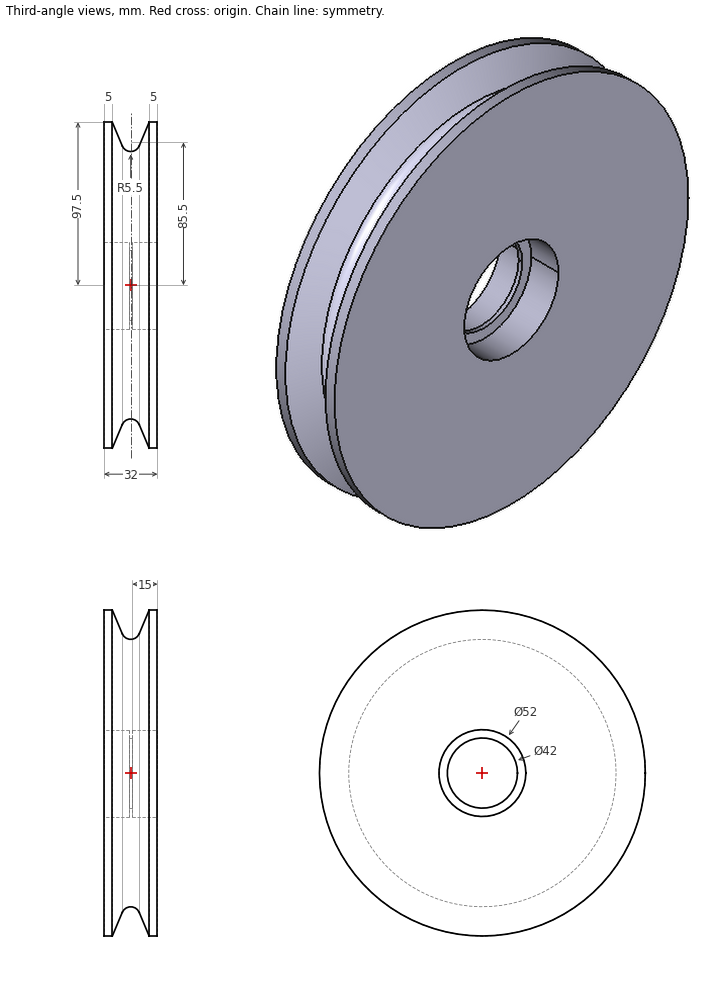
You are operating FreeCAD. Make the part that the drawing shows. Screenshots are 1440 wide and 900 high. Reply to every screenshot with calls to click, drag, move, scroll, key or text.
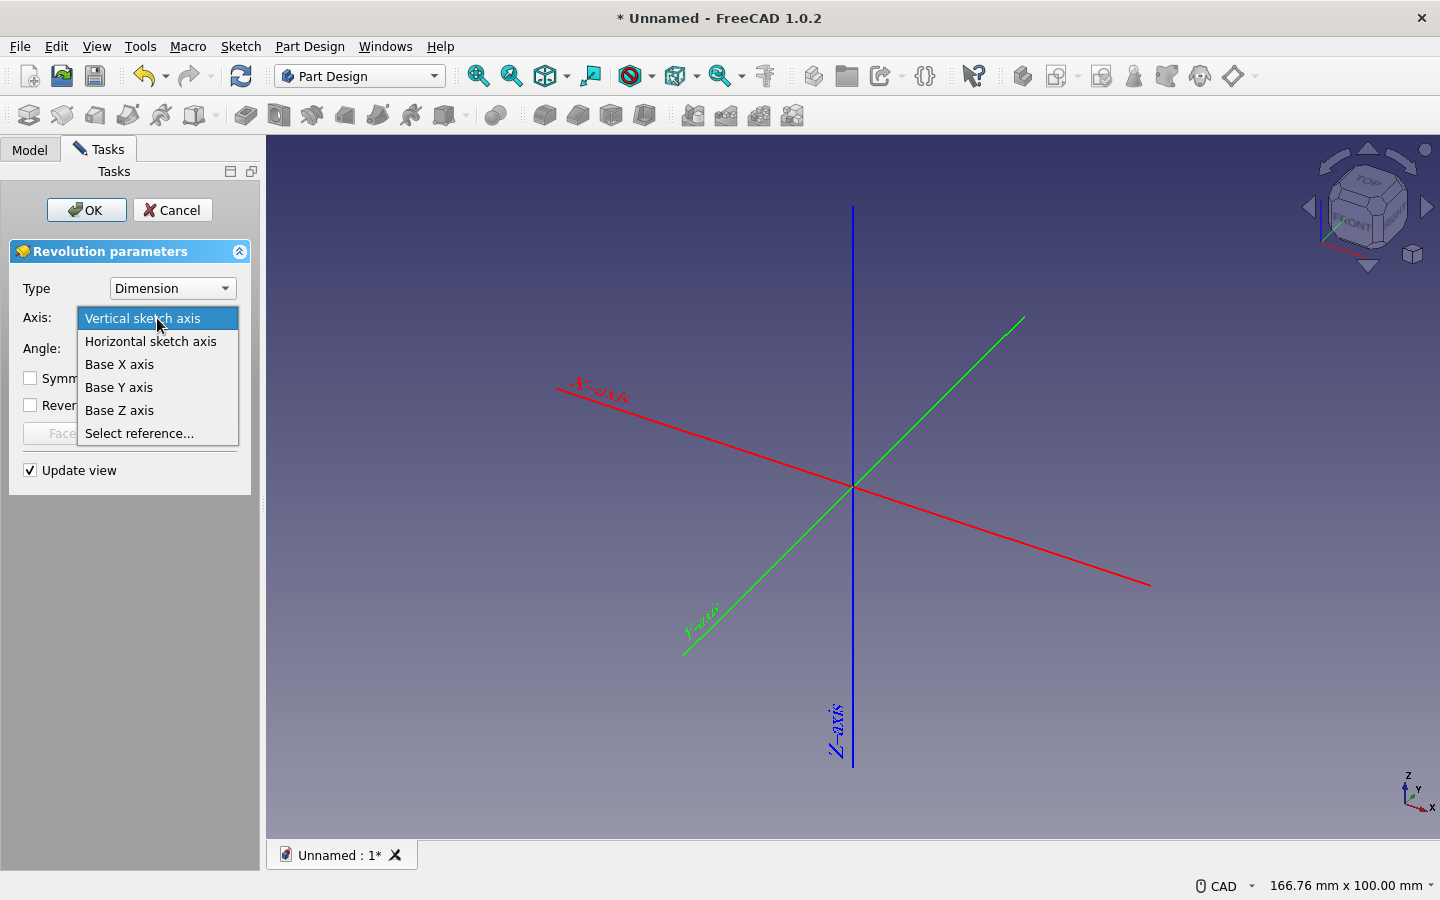
click(156, 342)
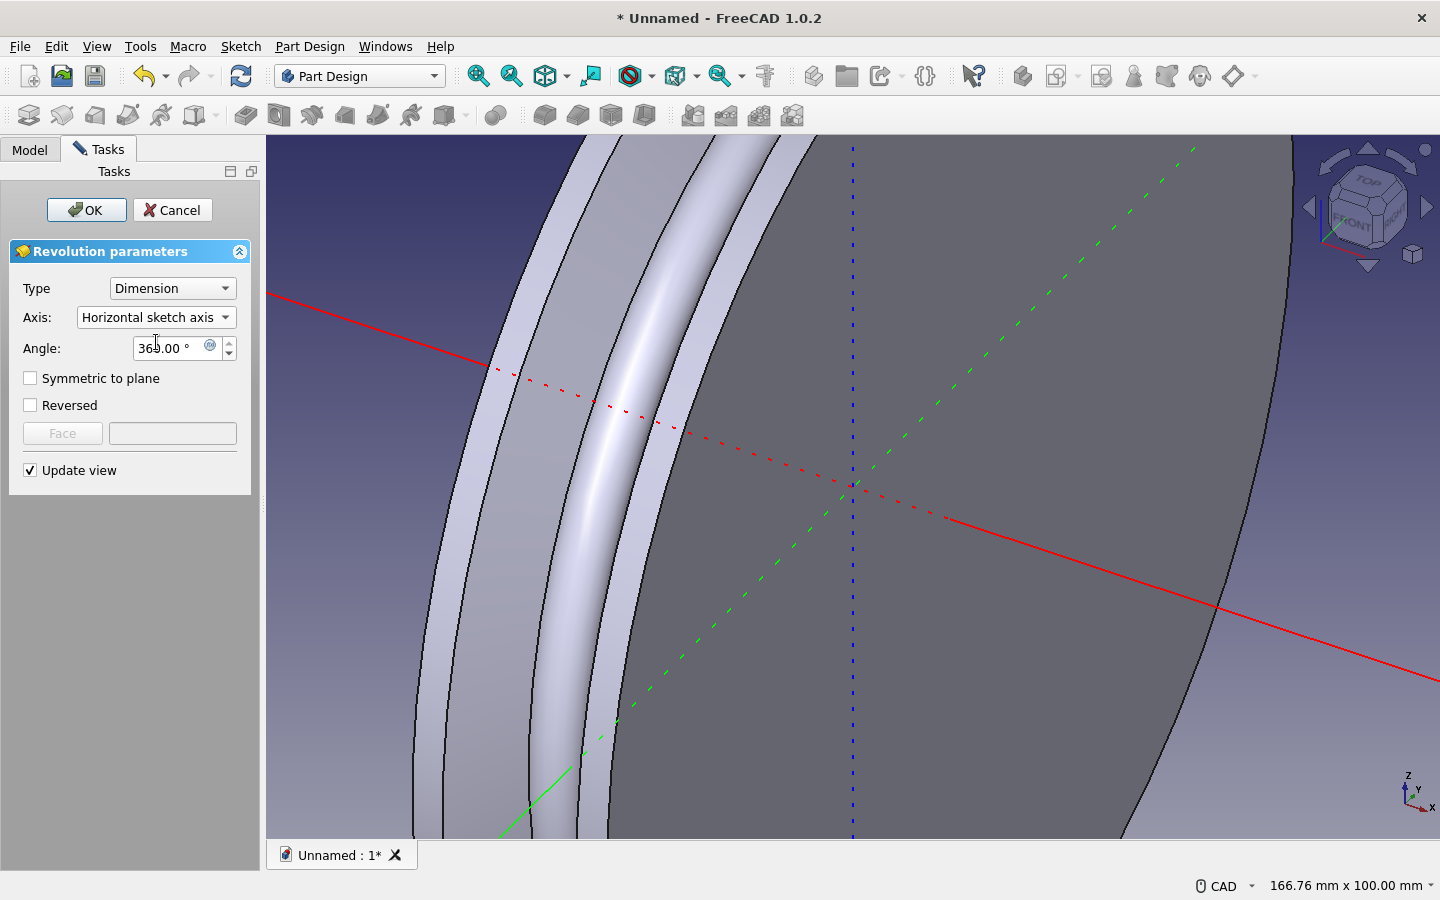
click(87, 210)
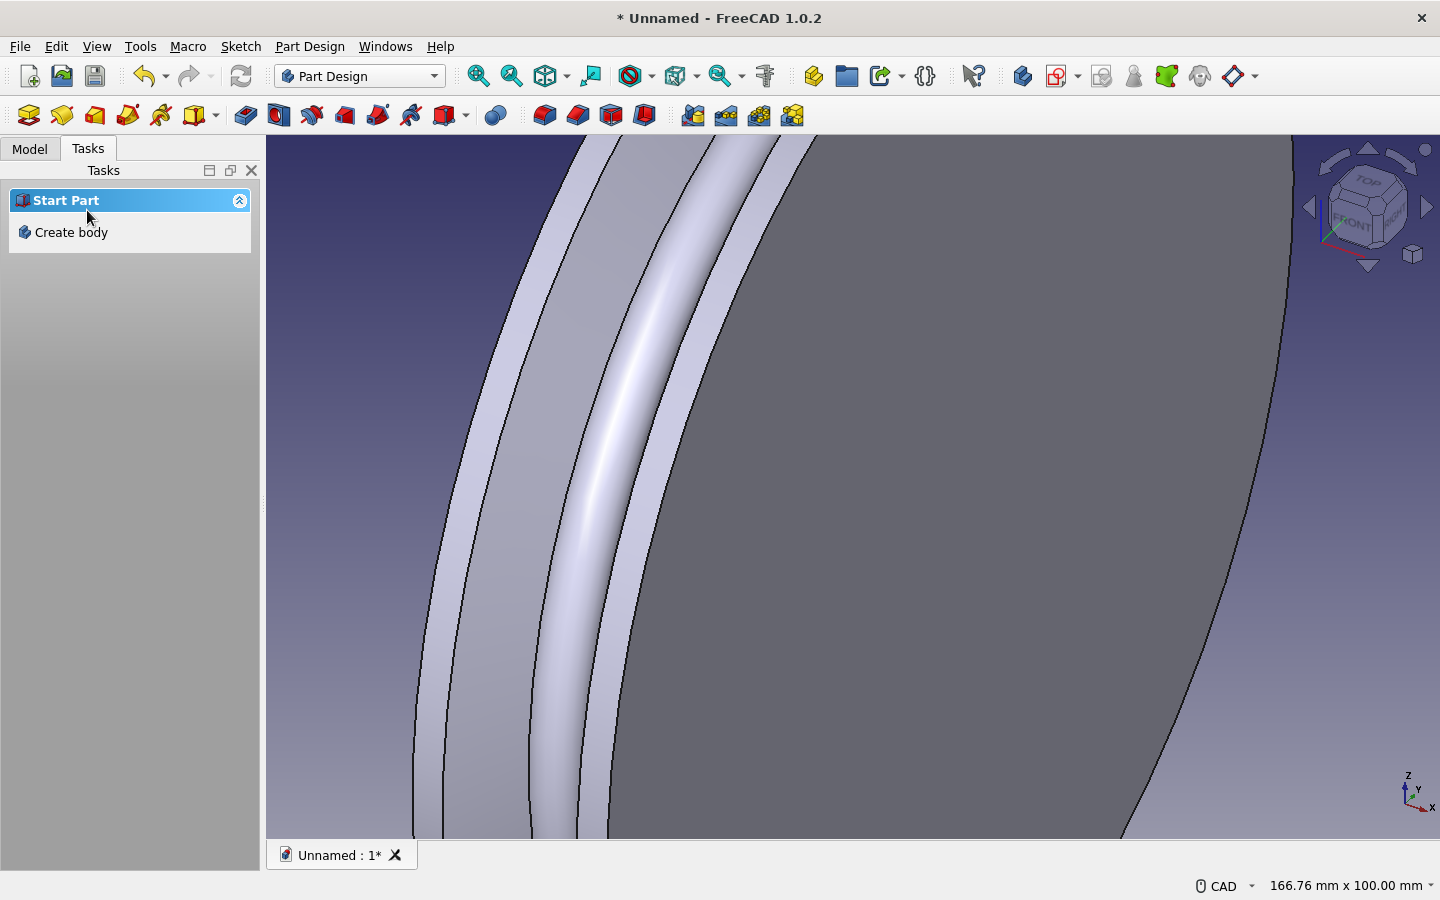
click(479, 76)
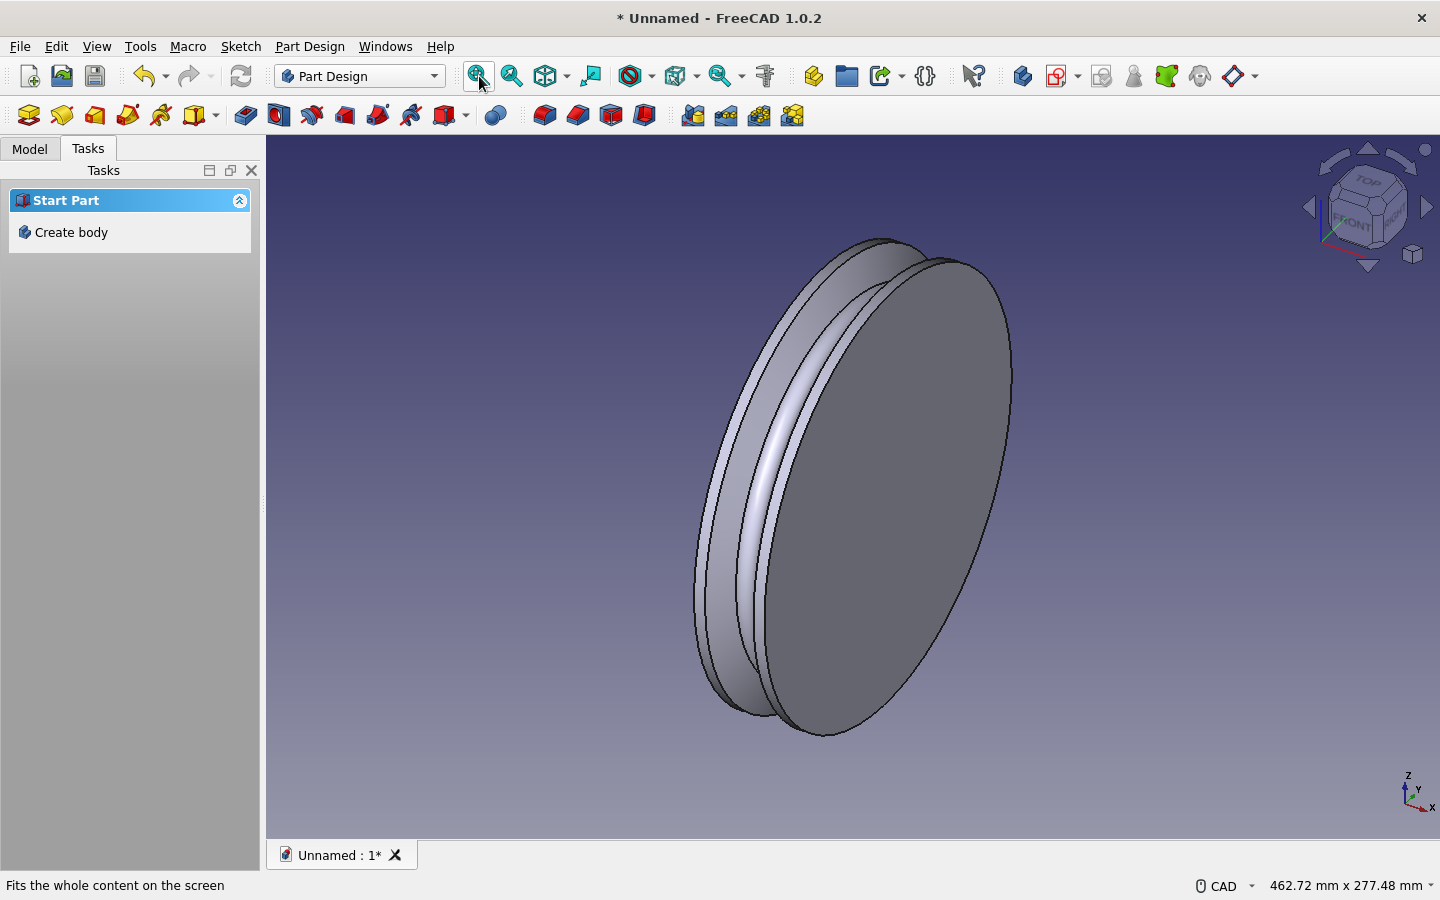
click(888, 498)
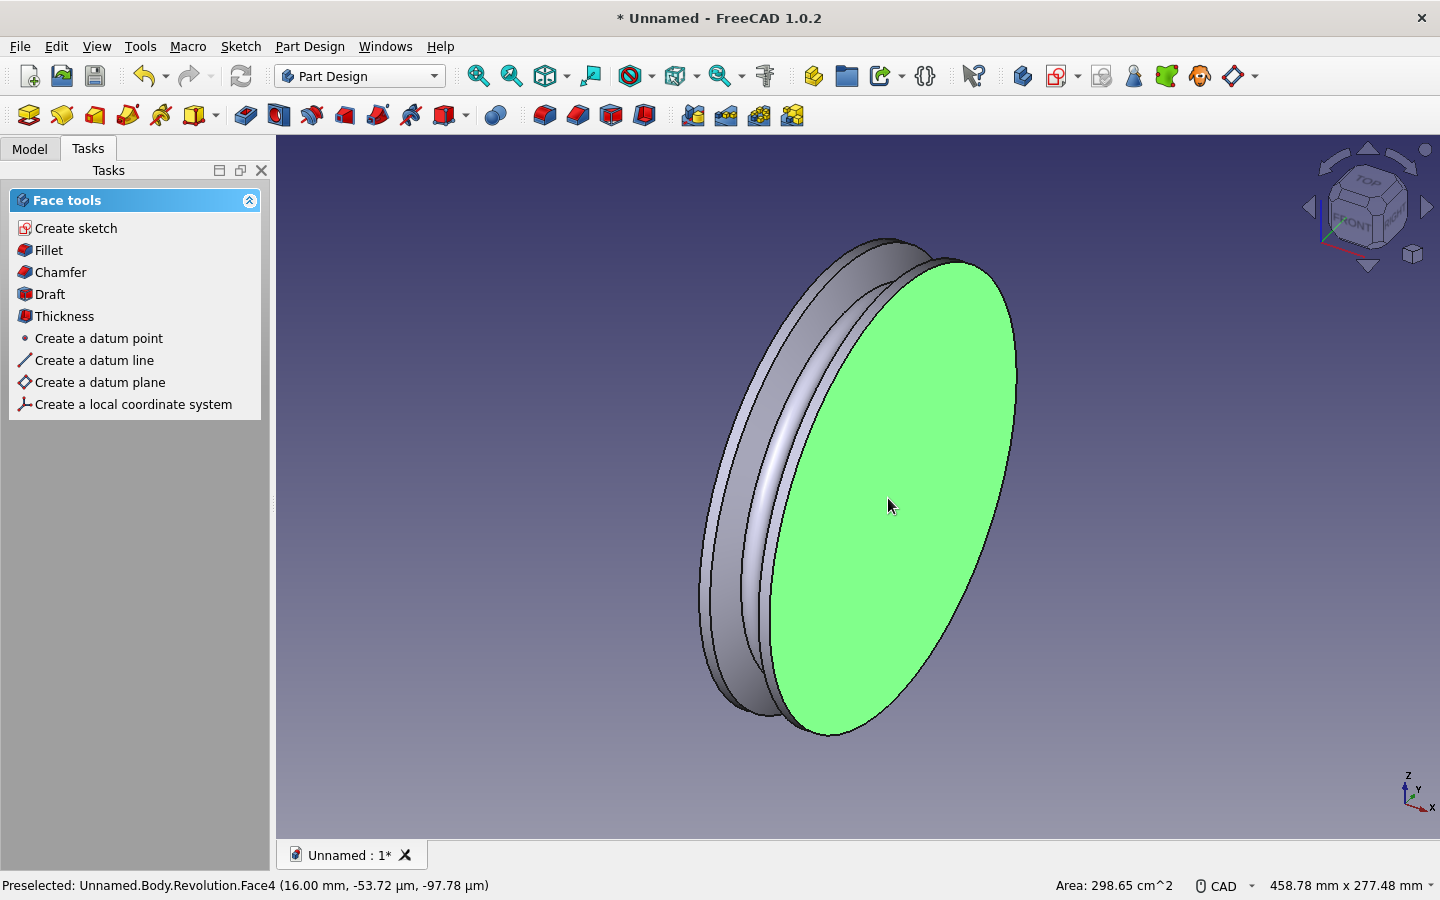
click(1056, 76)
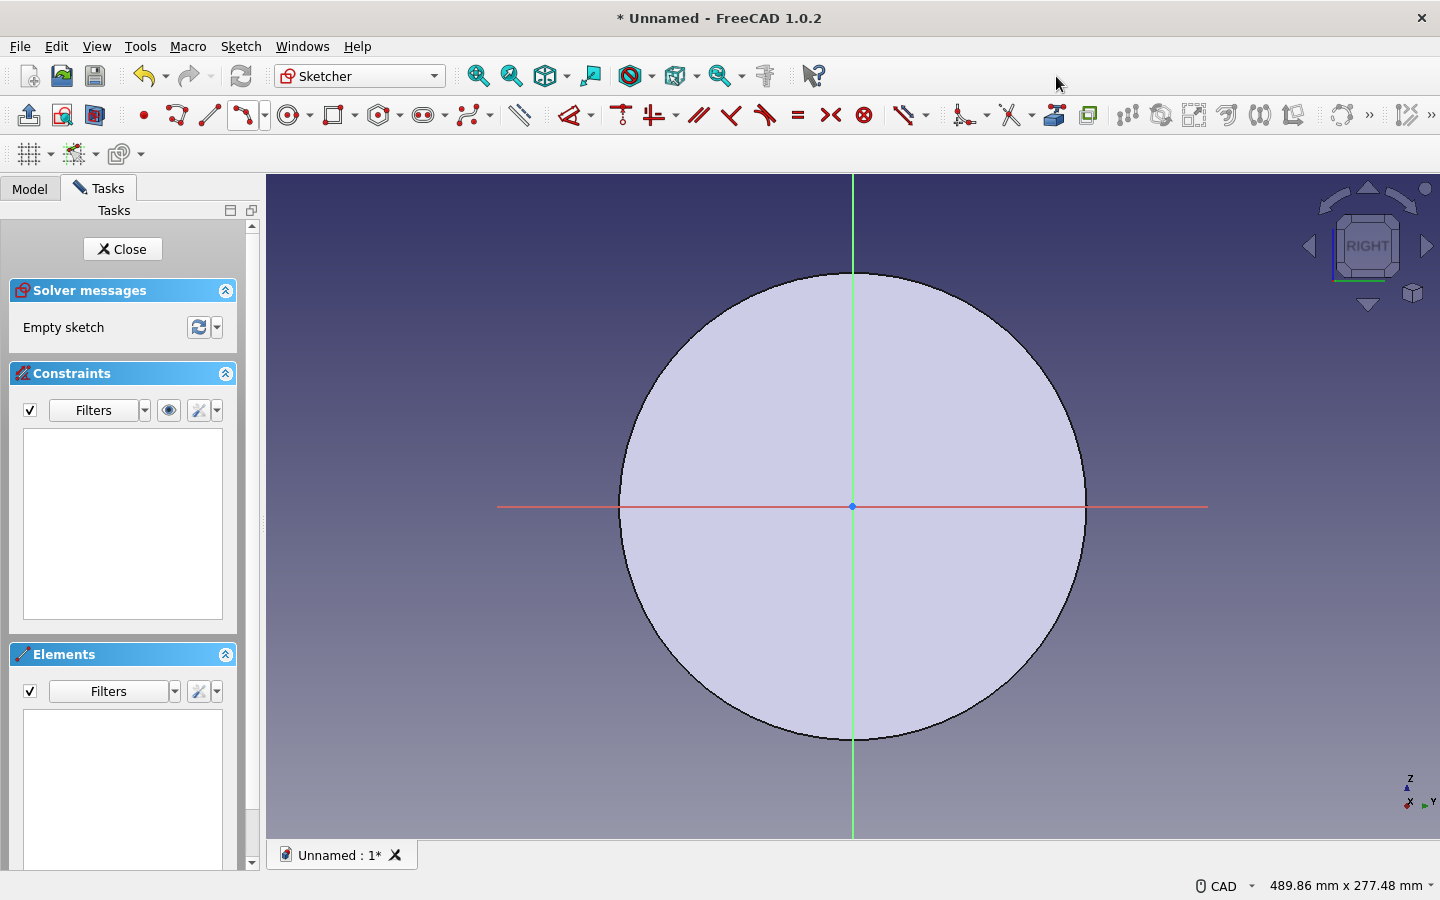
scroll(875, 507, up, 7)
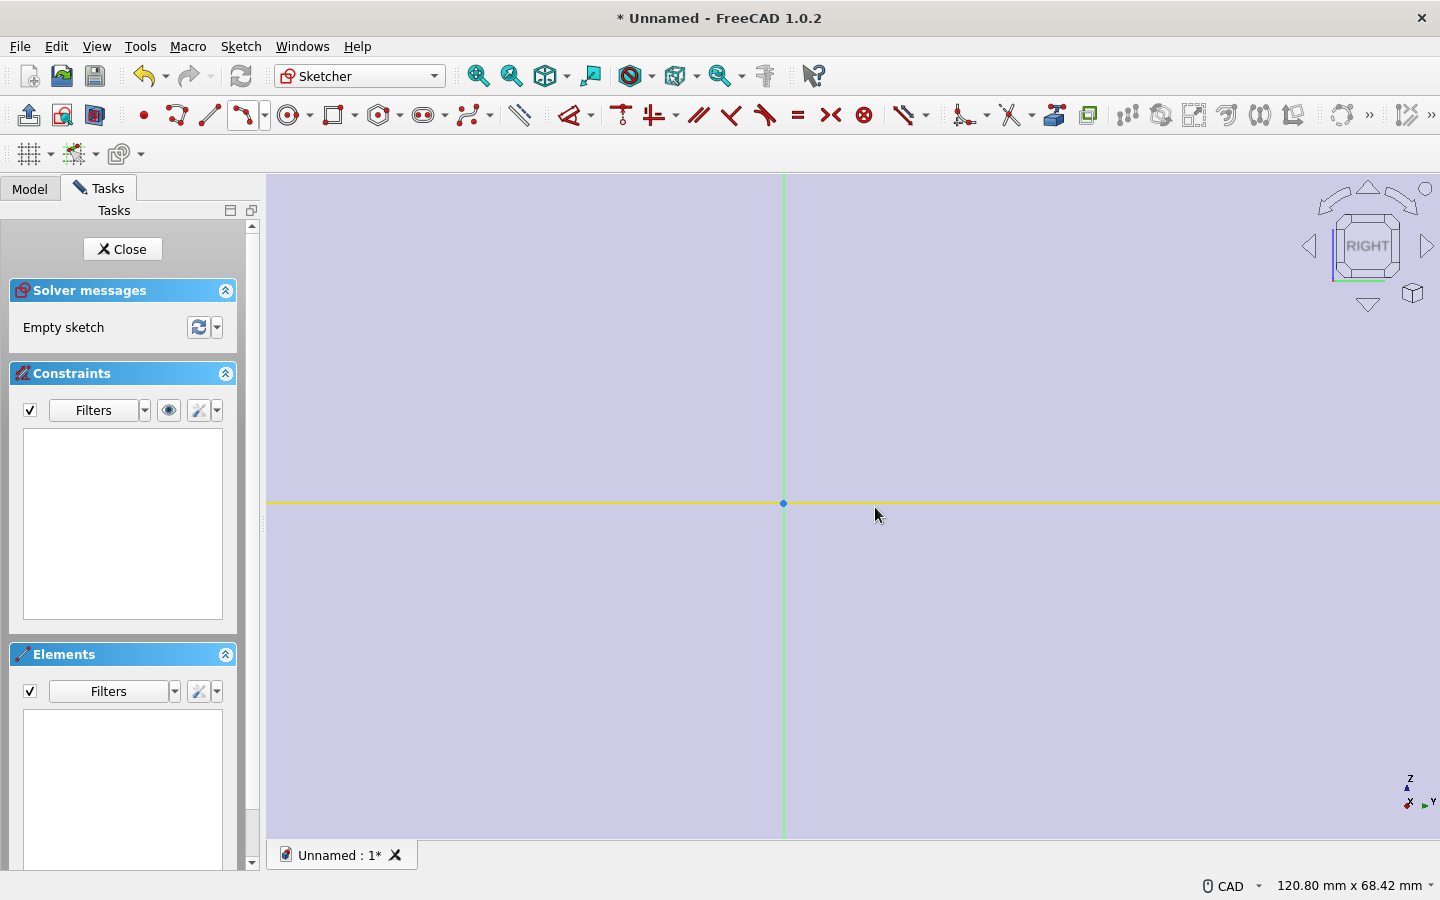
click(288, 116)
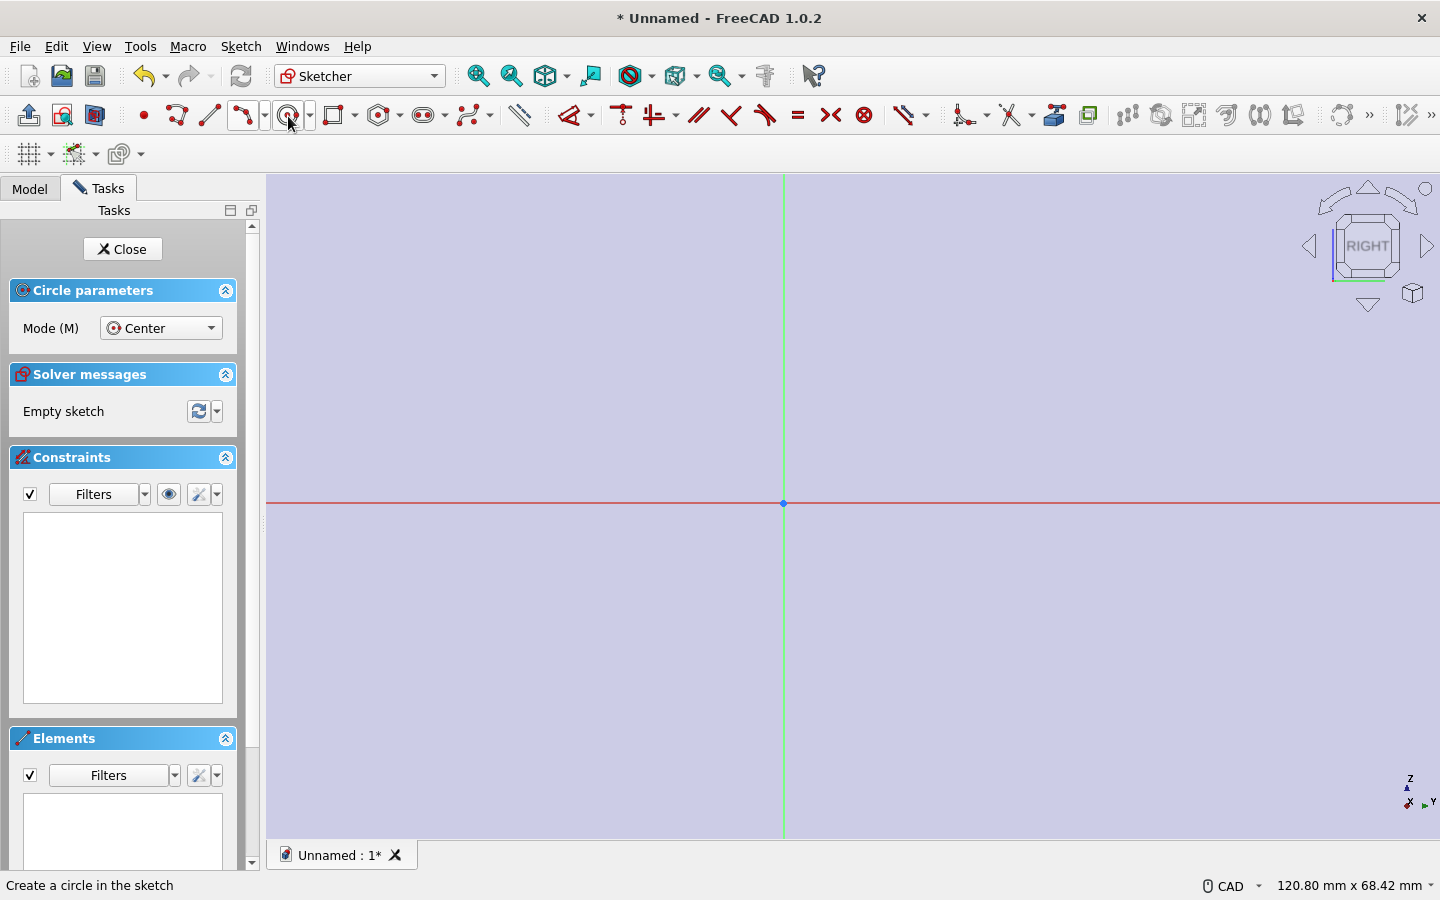
click(784, 503)
click(928, 359)
key(Escape)